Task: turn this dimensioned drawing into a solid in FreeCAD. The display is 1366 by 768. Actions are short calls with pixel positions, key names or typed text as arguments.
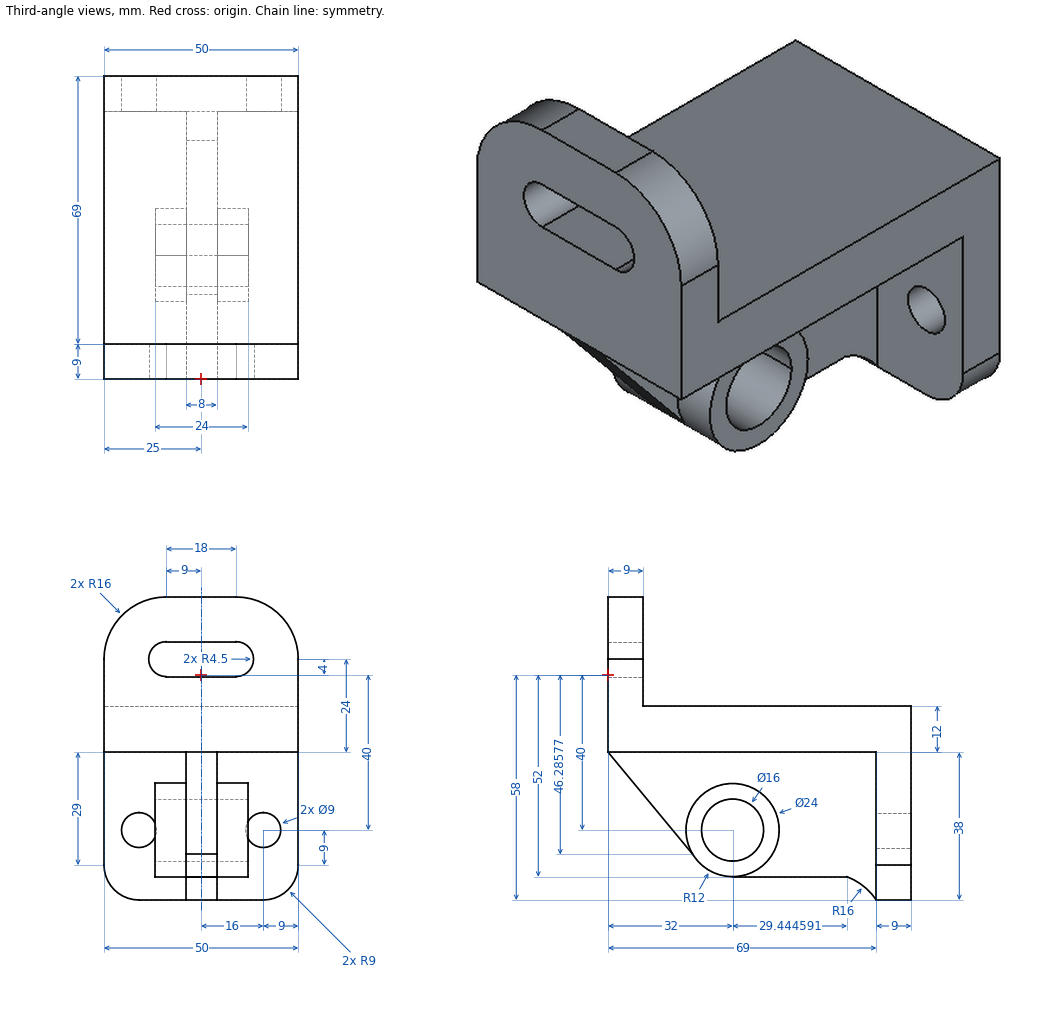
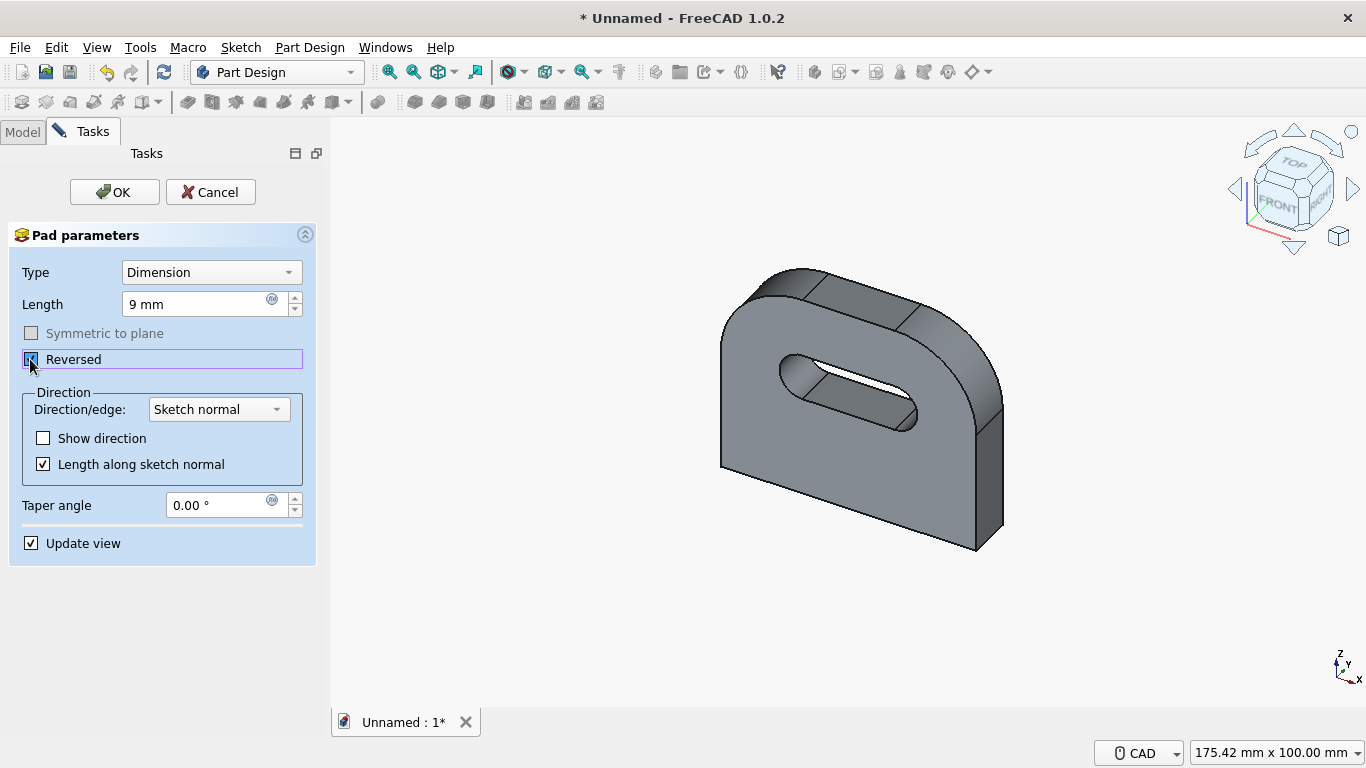
click(115, 192)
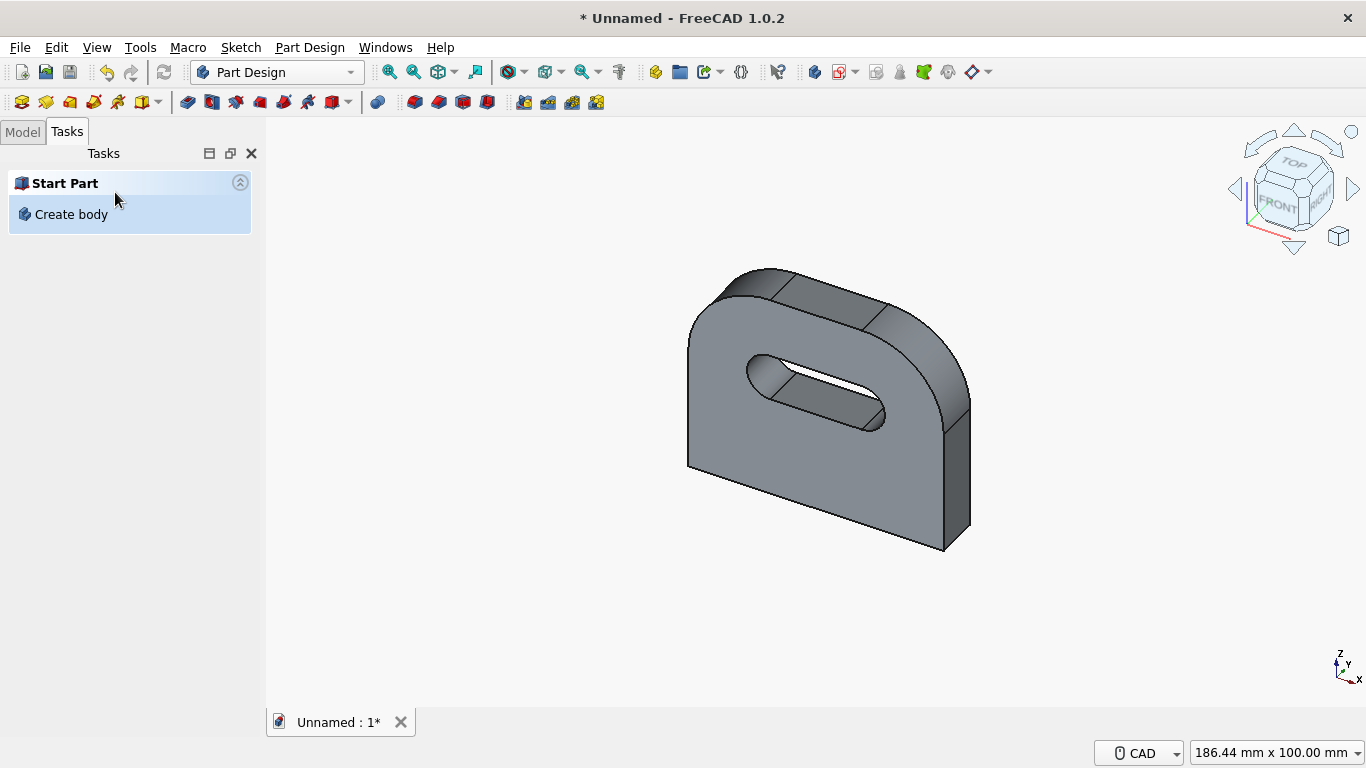
key(5)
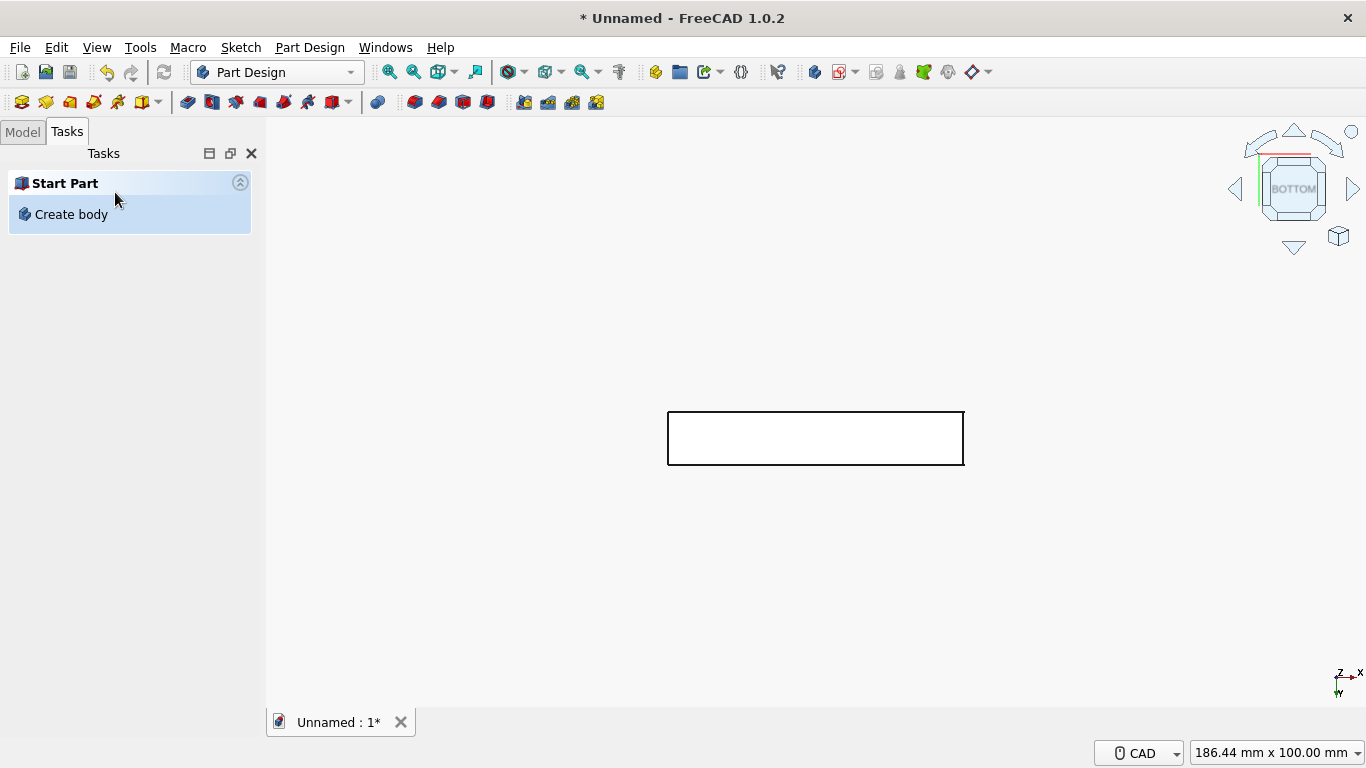
key(v)
key(f)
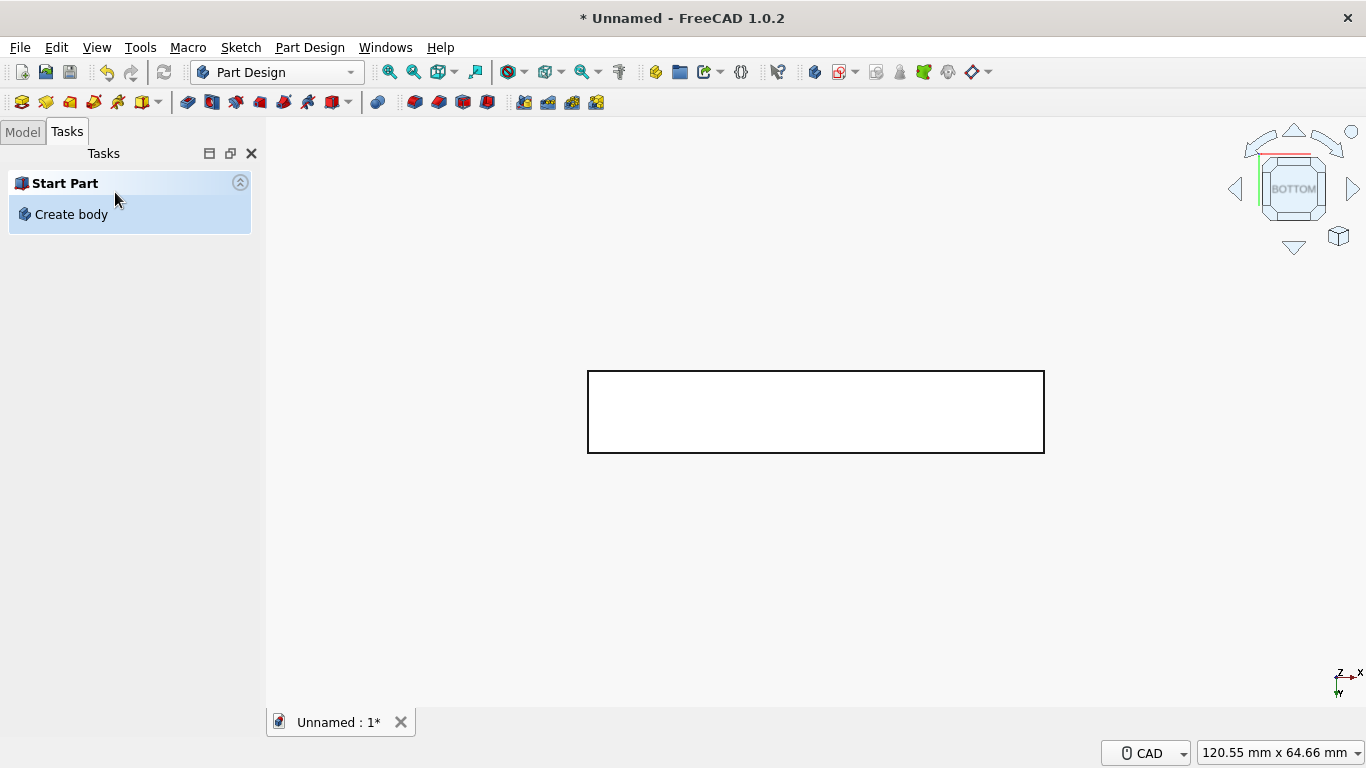
click(946, 411)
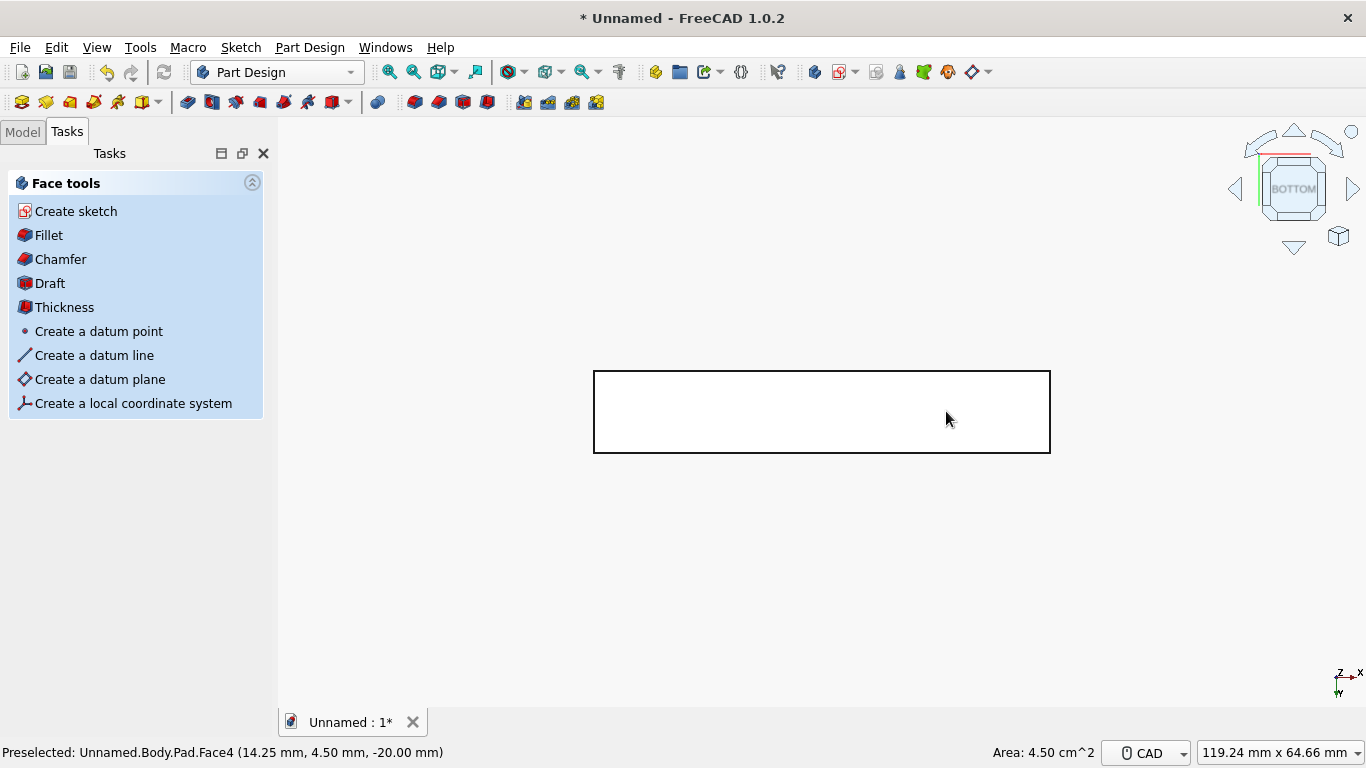
click(840, 72)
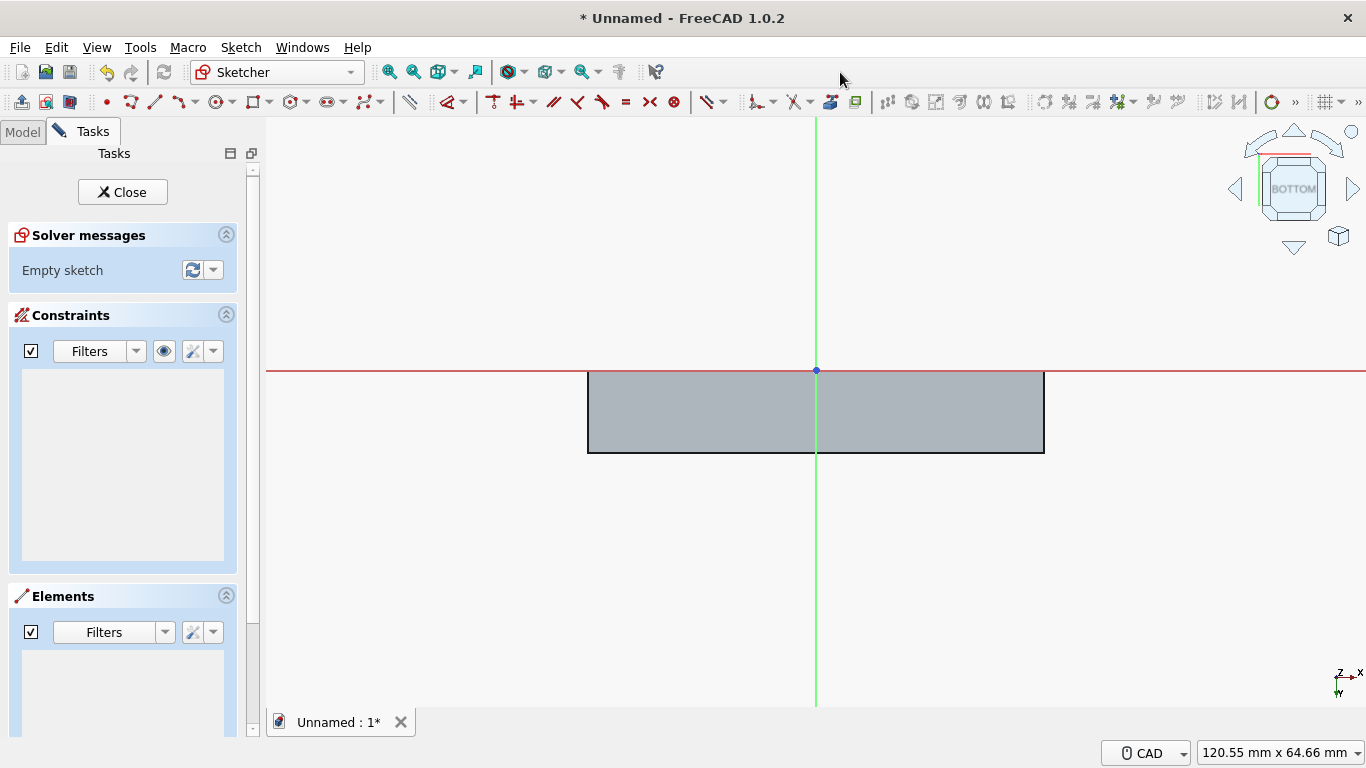
scroll(692, 155, down, 4)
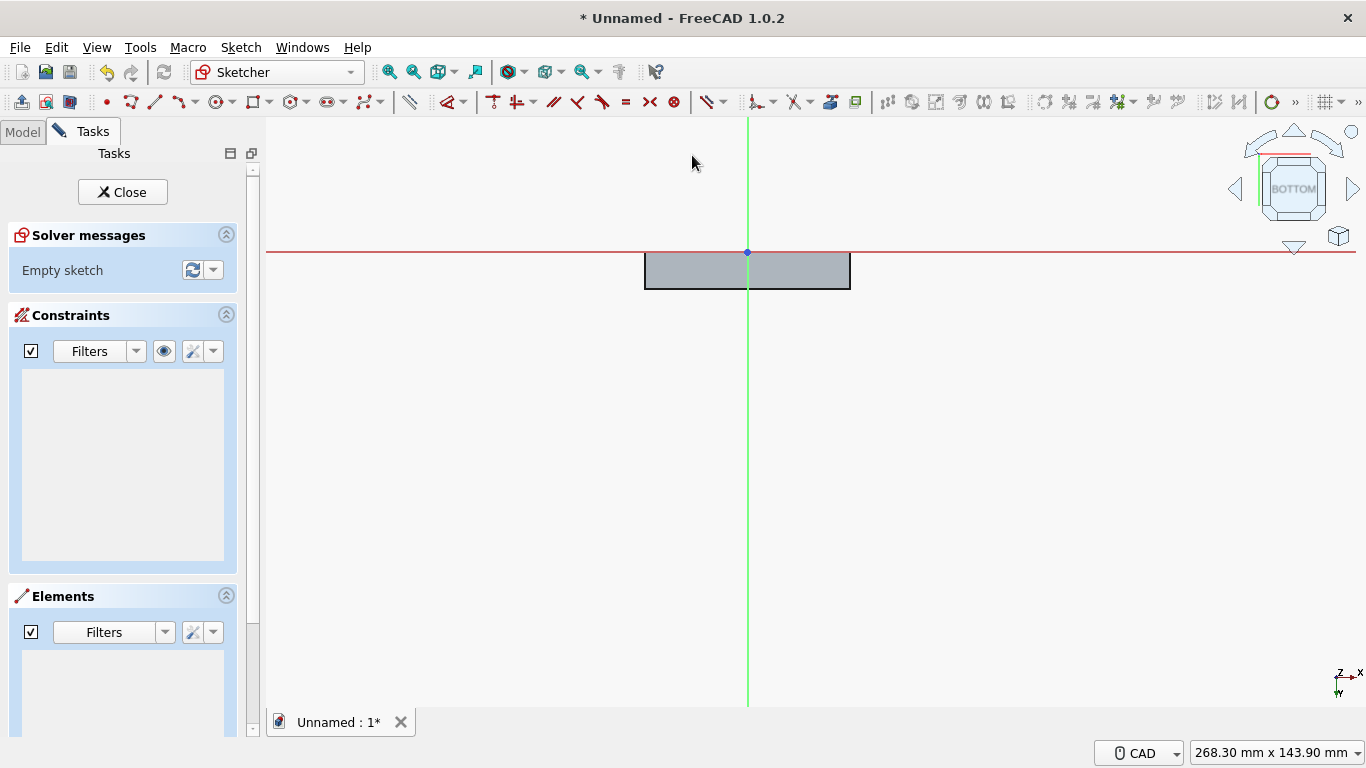
click(254, 102)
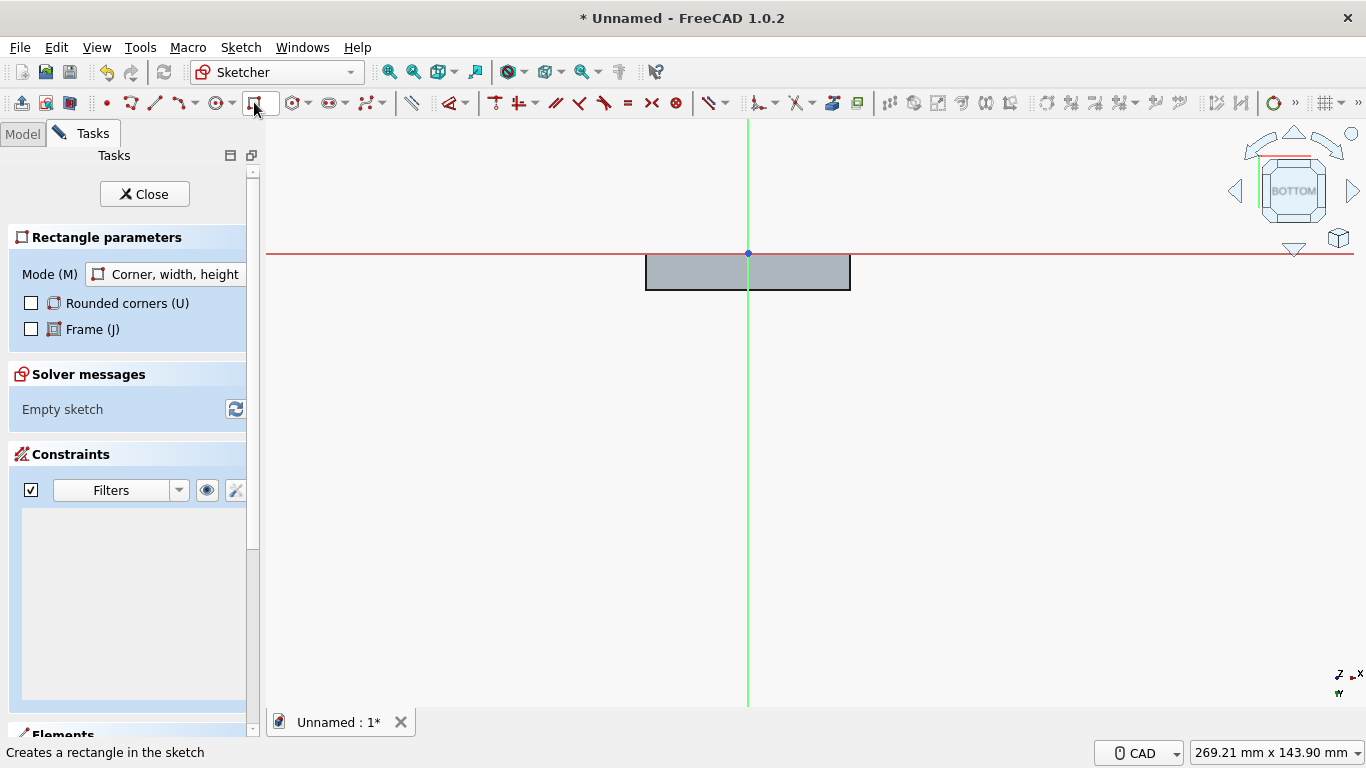
click(646, 290)
click(850, 572)
key(Escape)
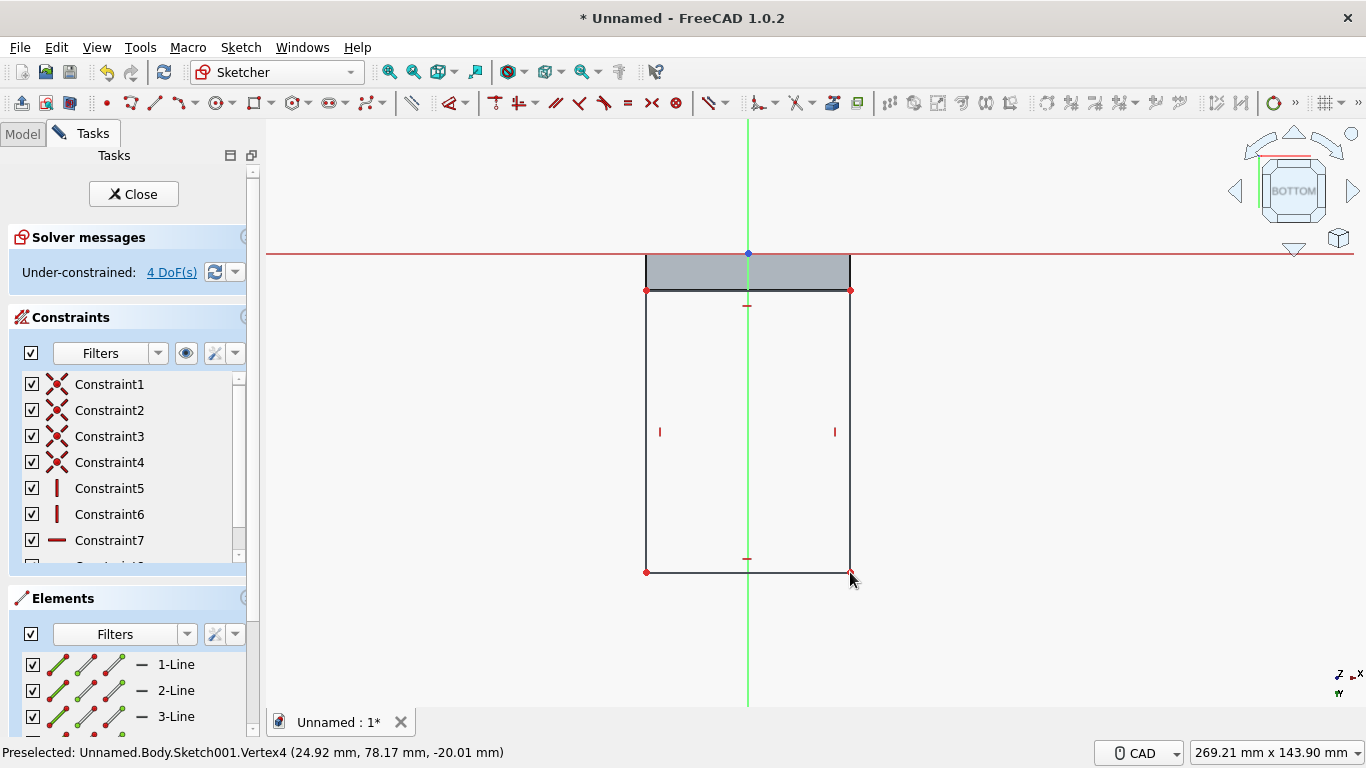
click(450, 104)